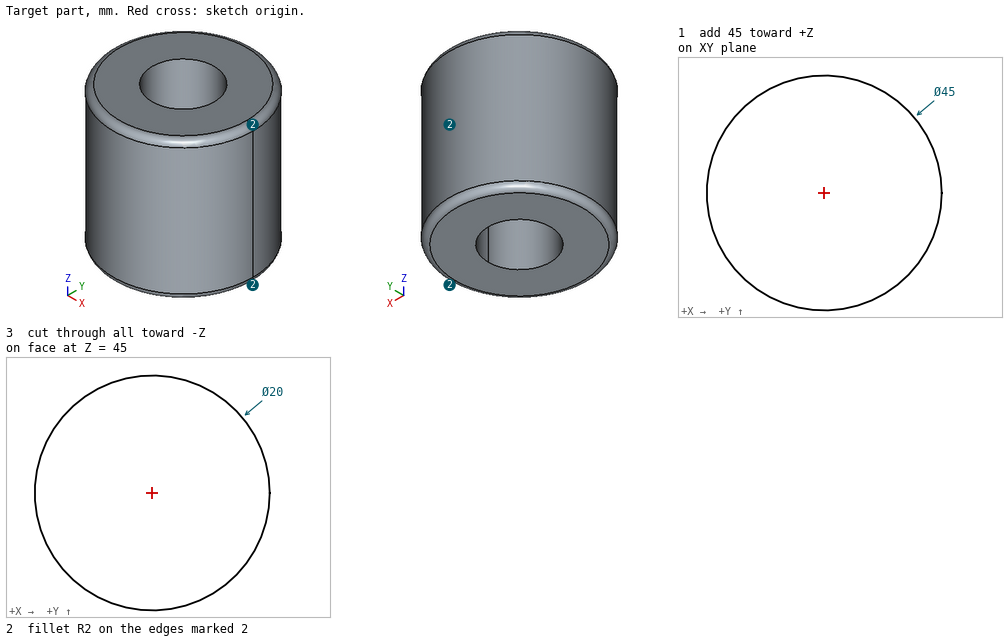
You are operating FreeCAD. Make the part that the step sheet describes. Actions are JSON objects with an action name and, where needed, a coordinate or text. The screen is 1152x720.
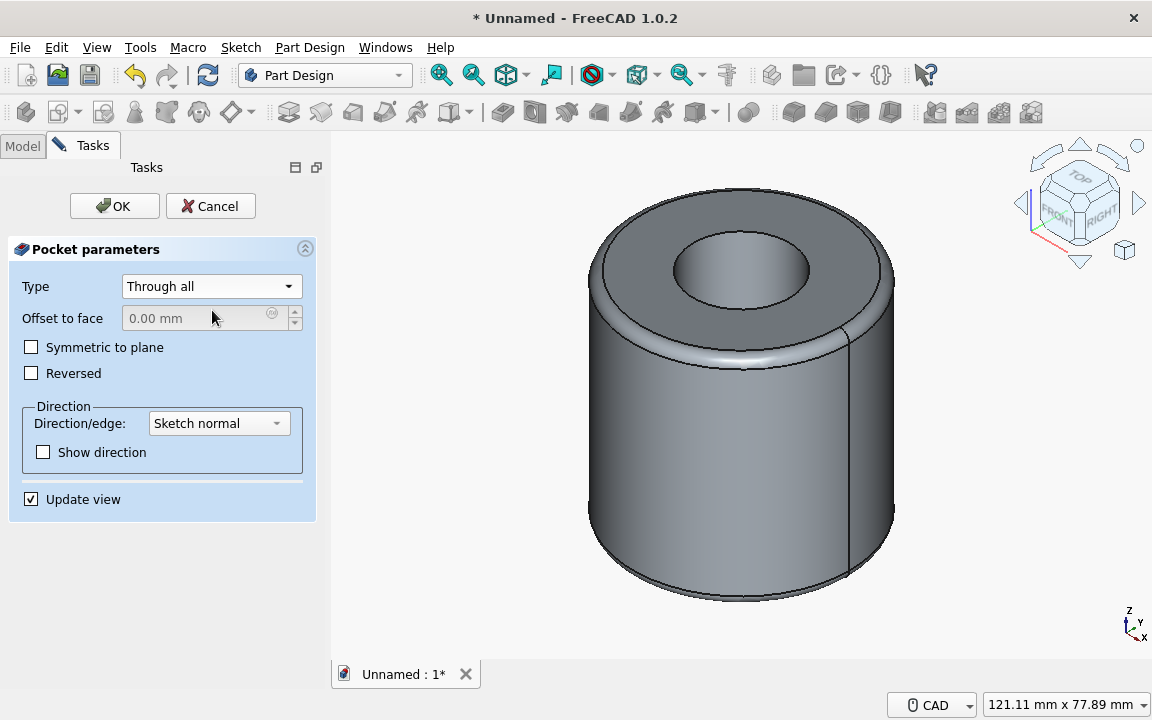
{"action": "left_click", "coordinate": [115, 206]}